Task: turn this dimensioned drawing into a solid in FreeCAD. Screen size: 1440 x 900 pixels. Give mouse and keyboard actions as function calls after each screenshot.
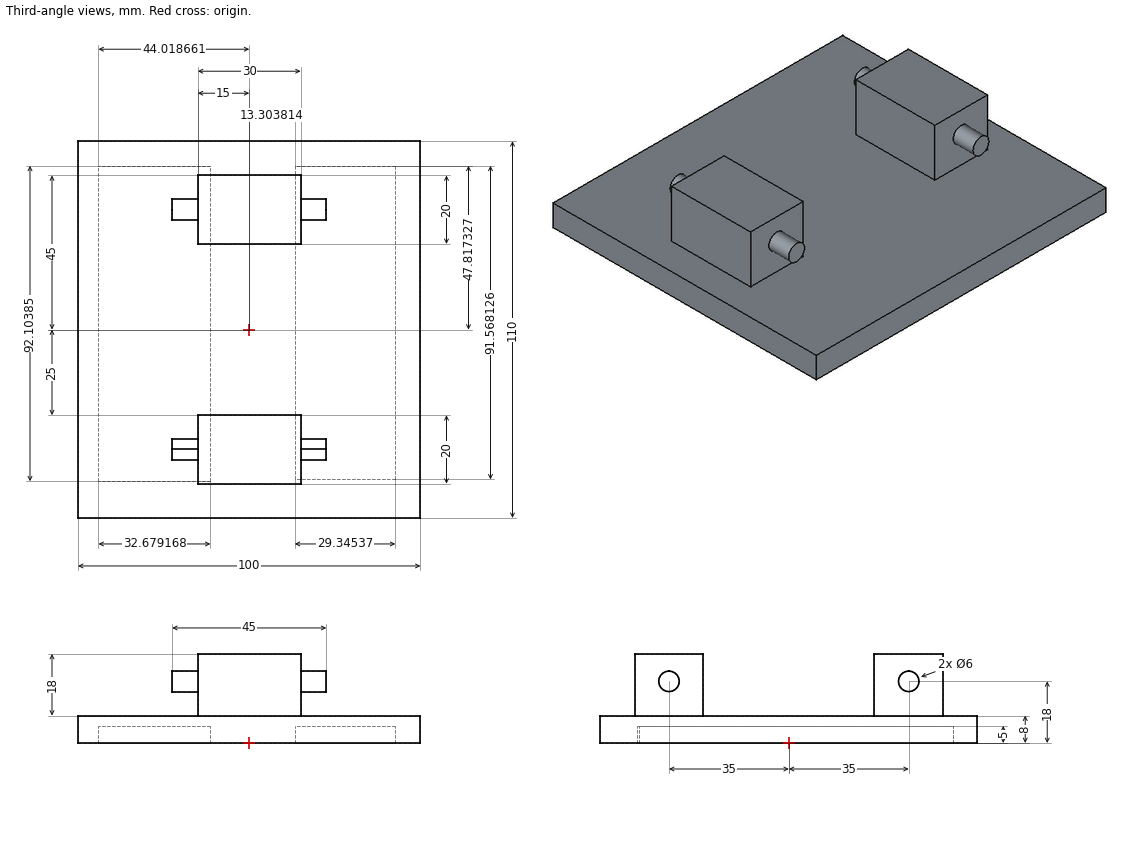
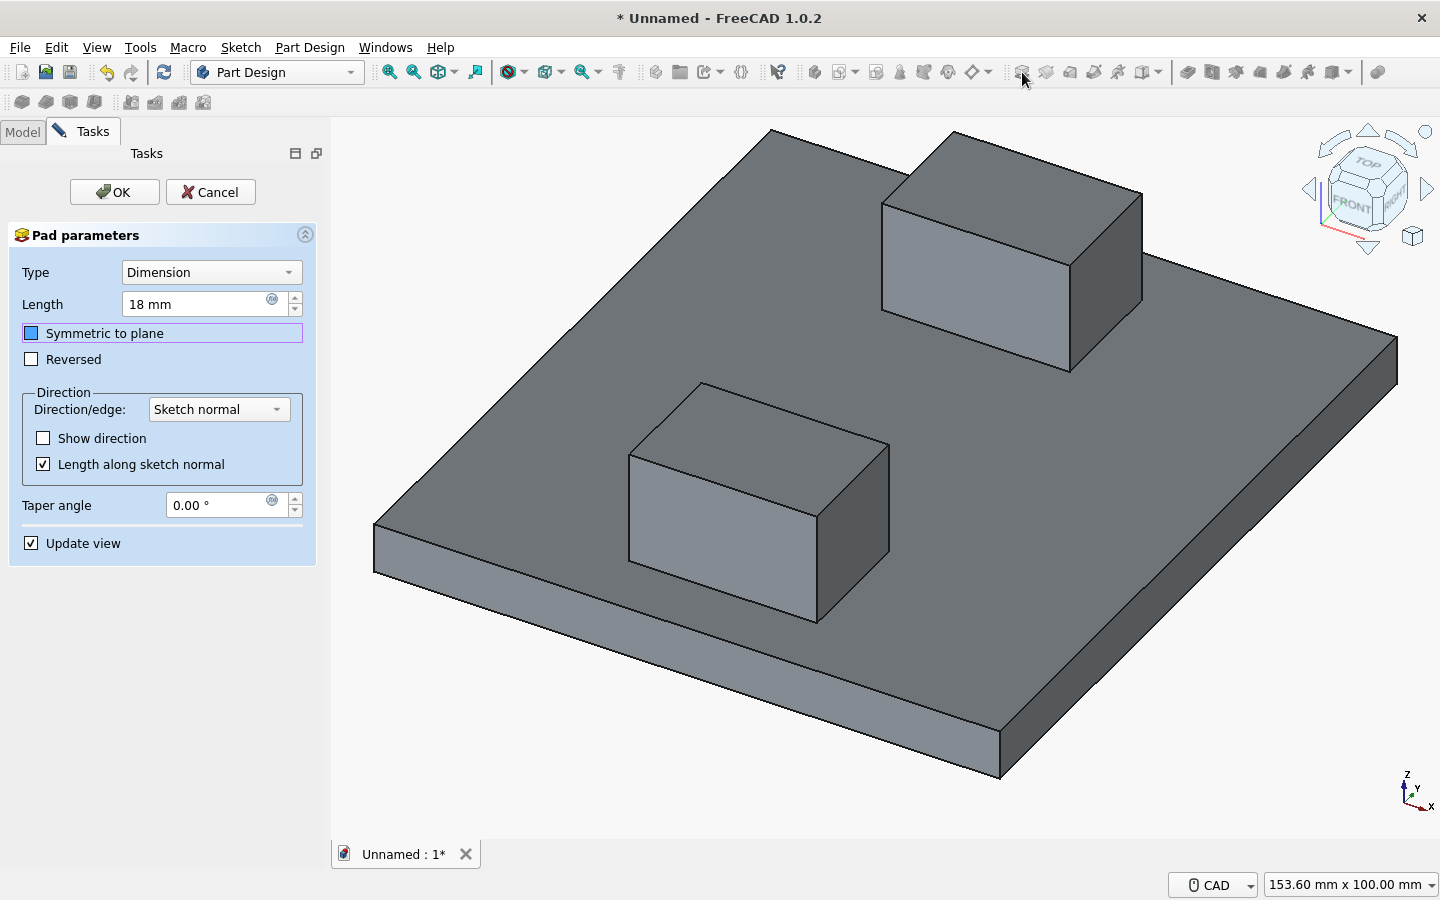
click(115, 192)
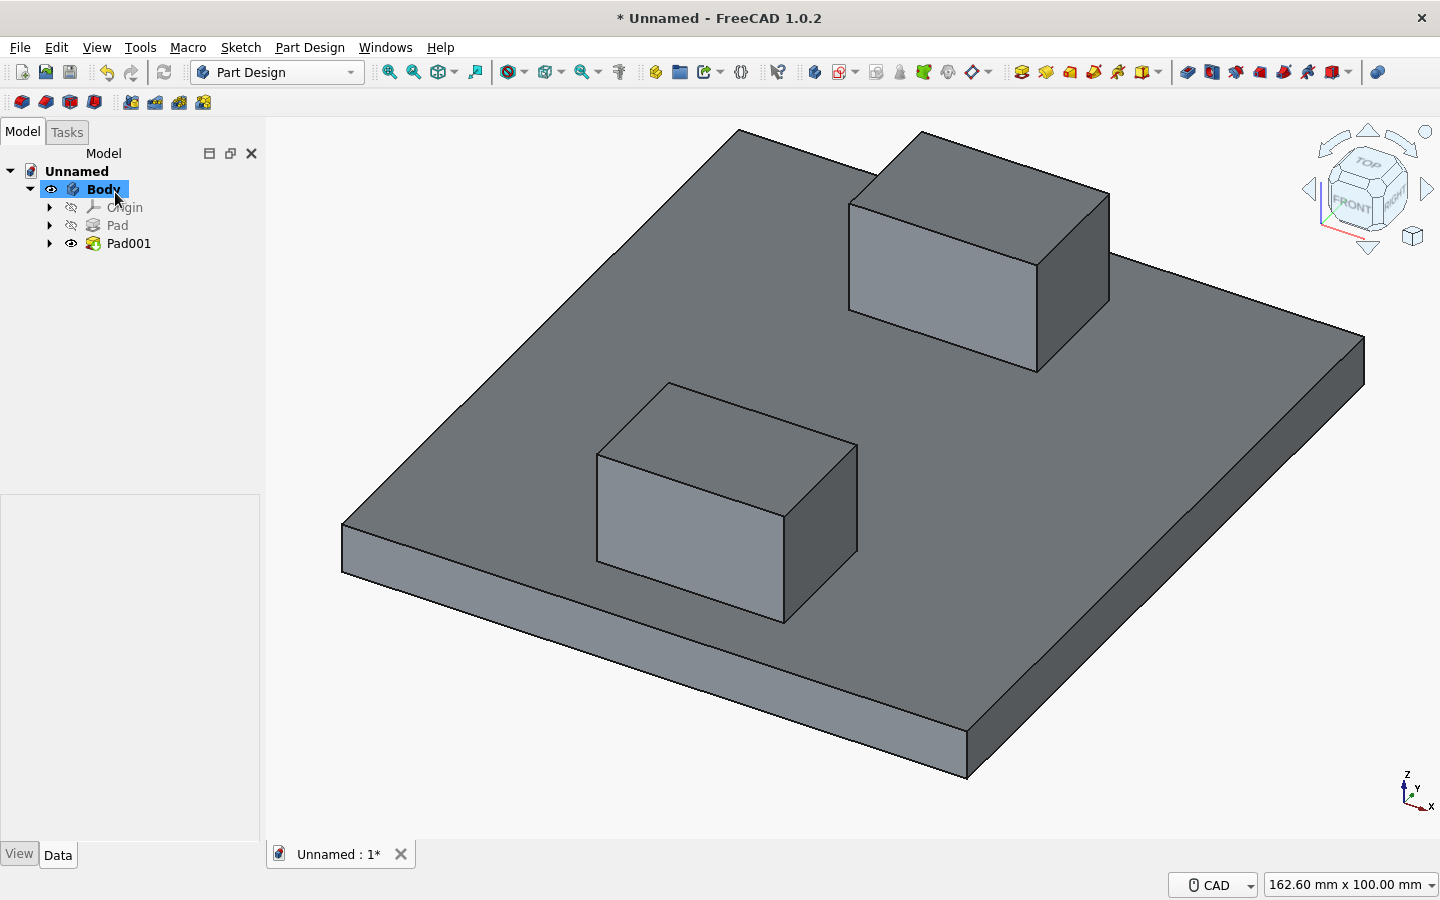
key(v)
key(f)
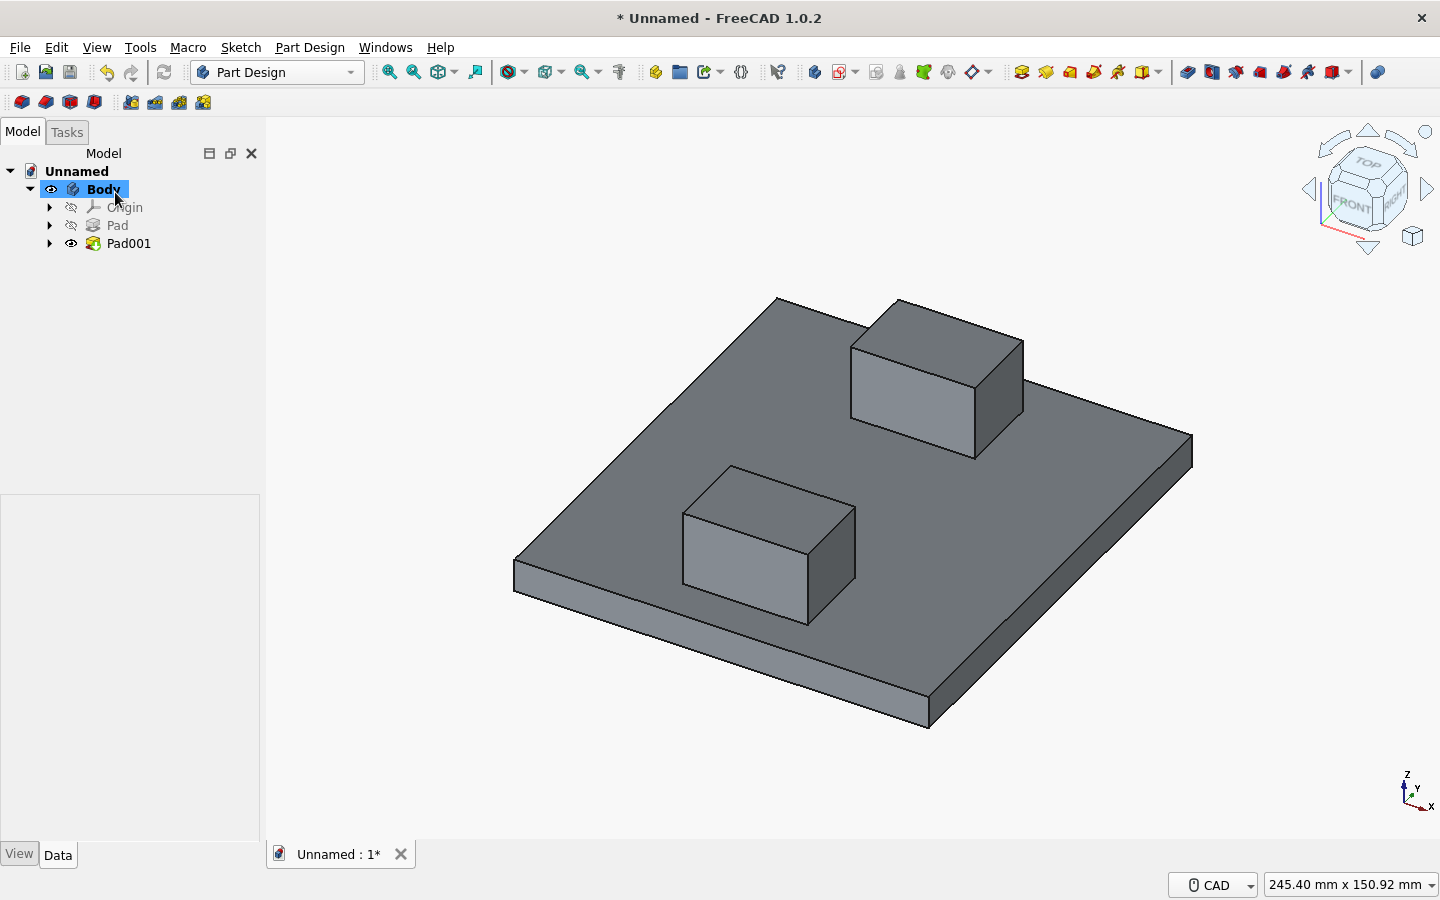
click(840, 72)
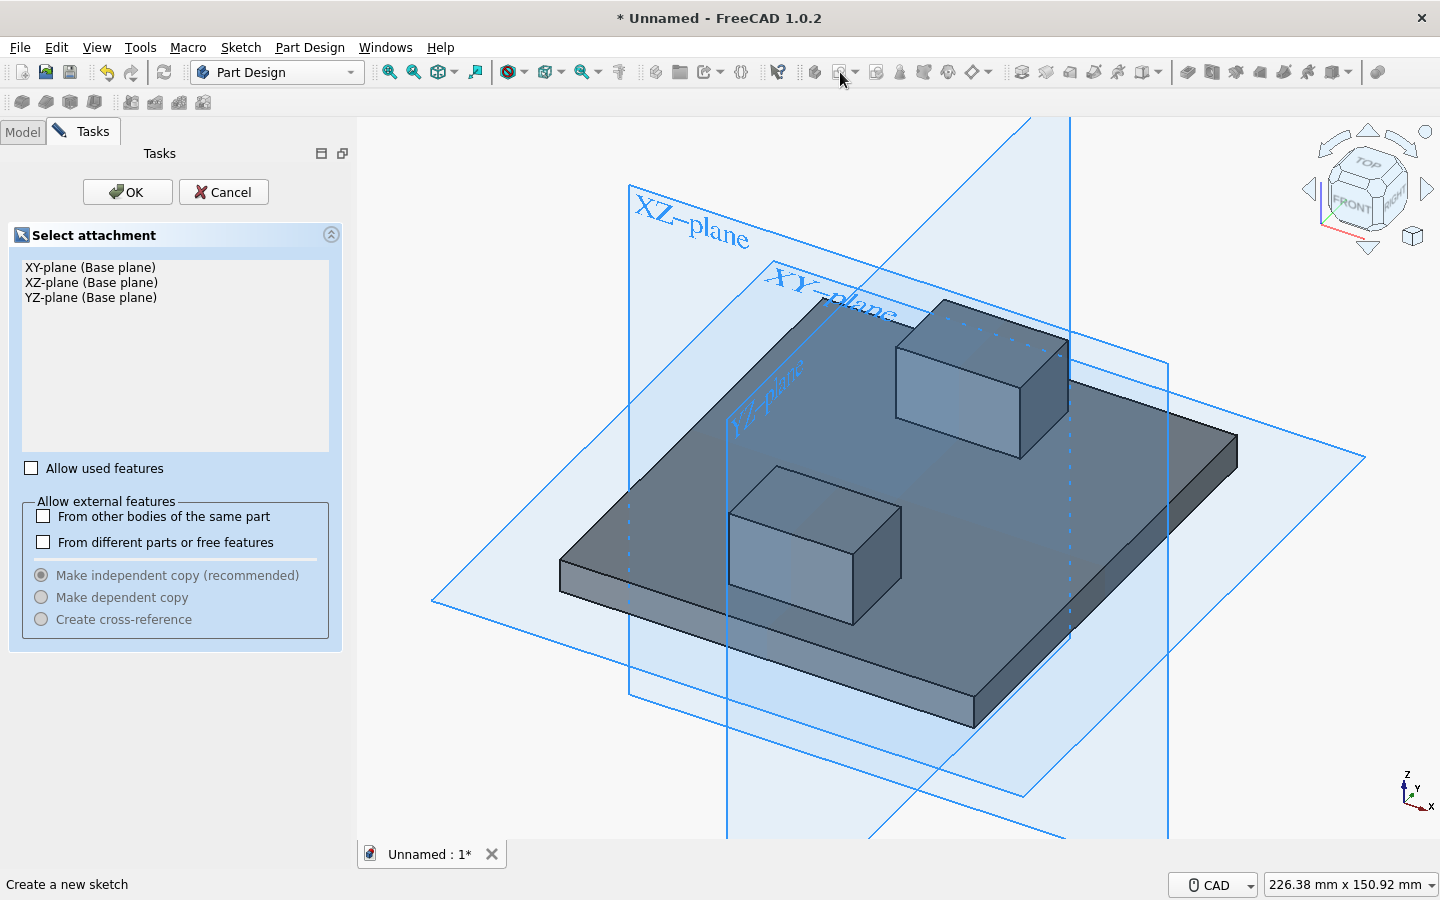
click(82, 268)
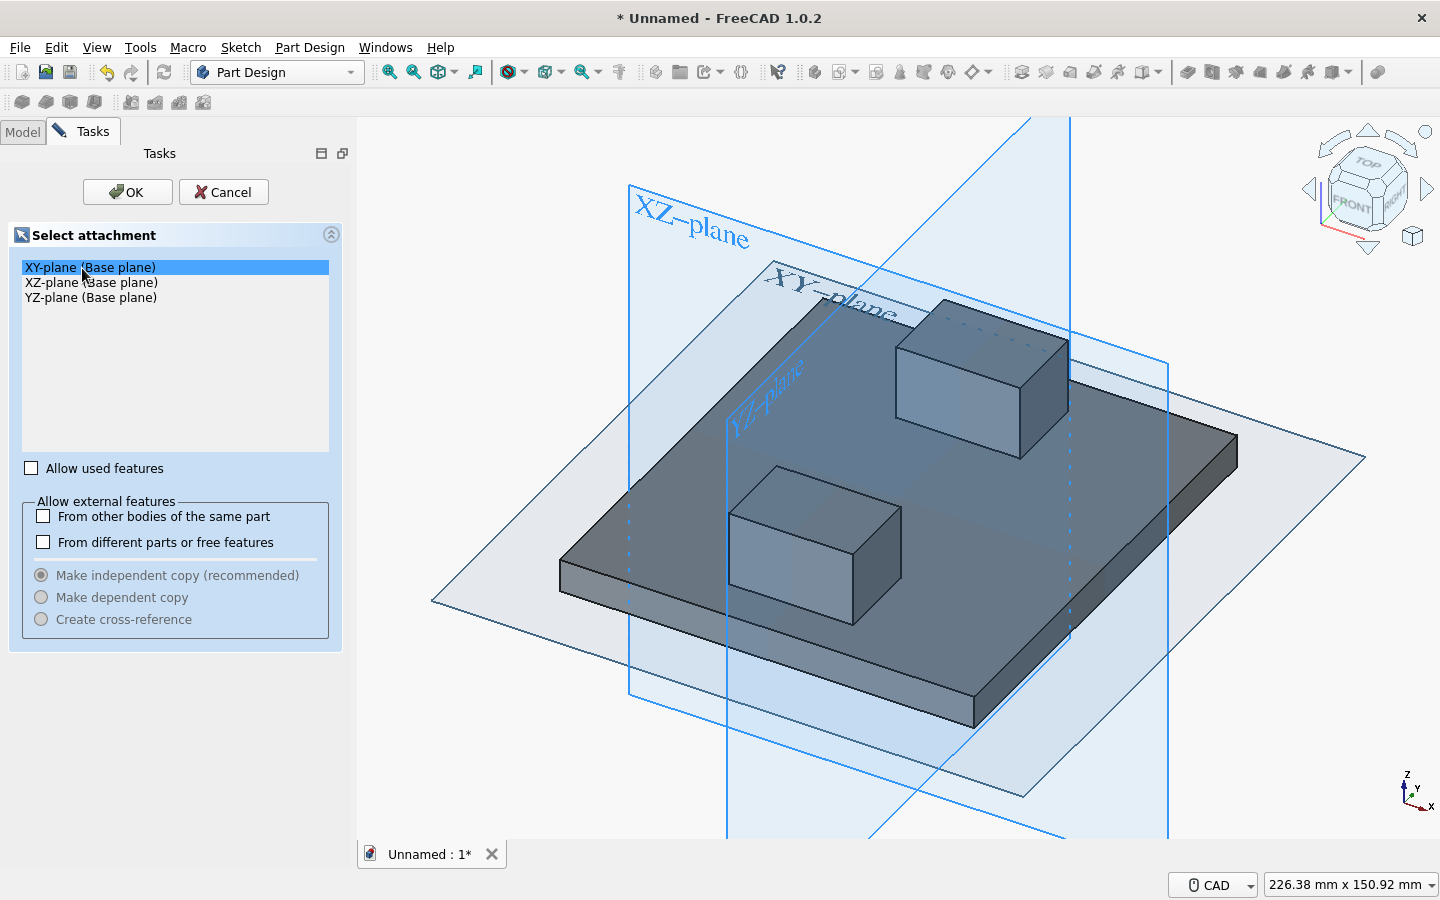
click(128, 192)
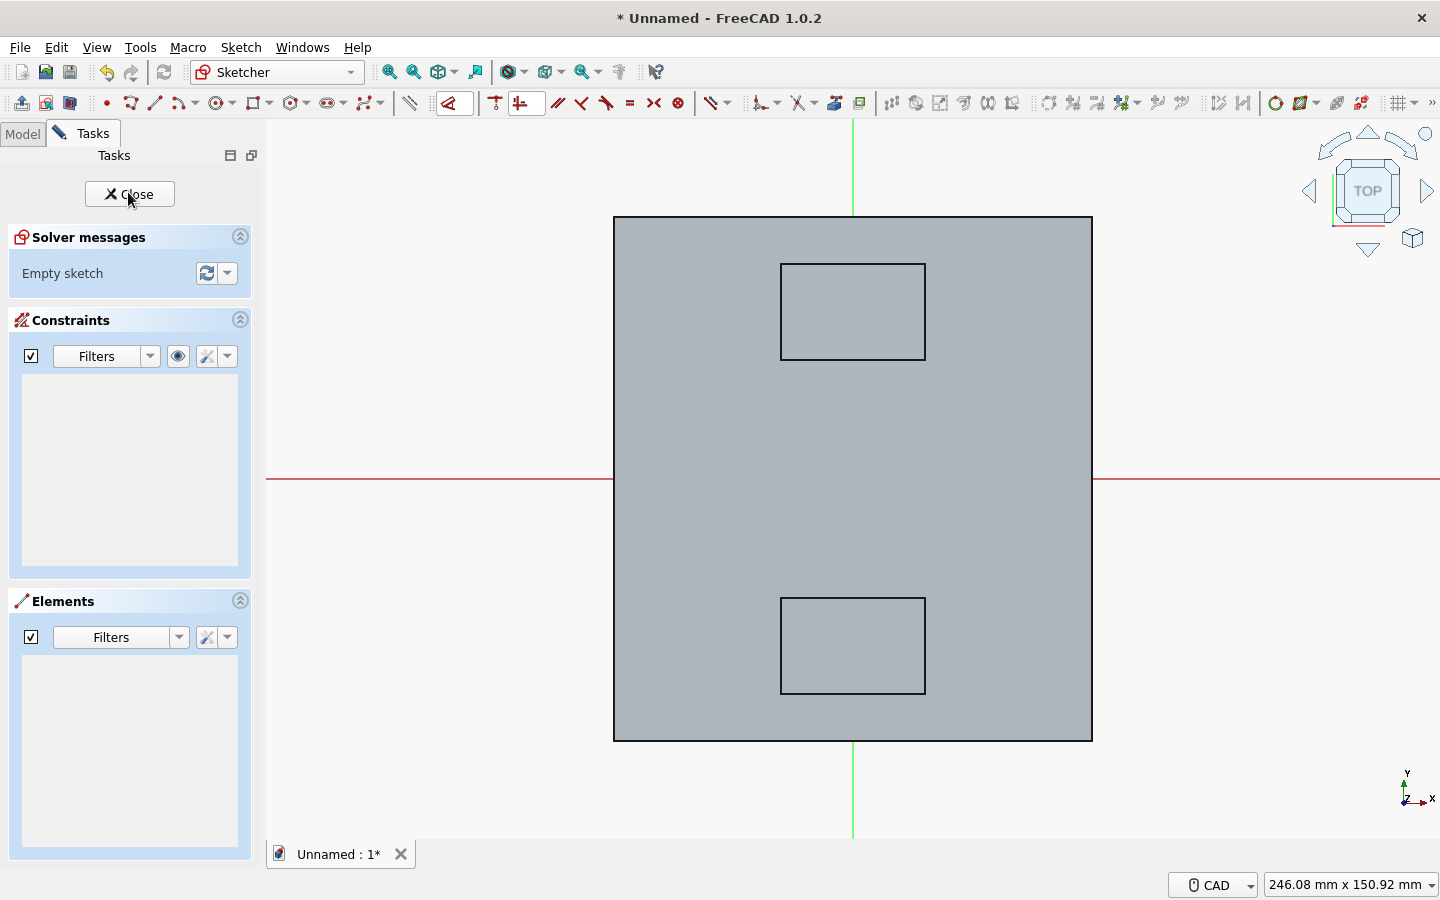
key(q)
key(s)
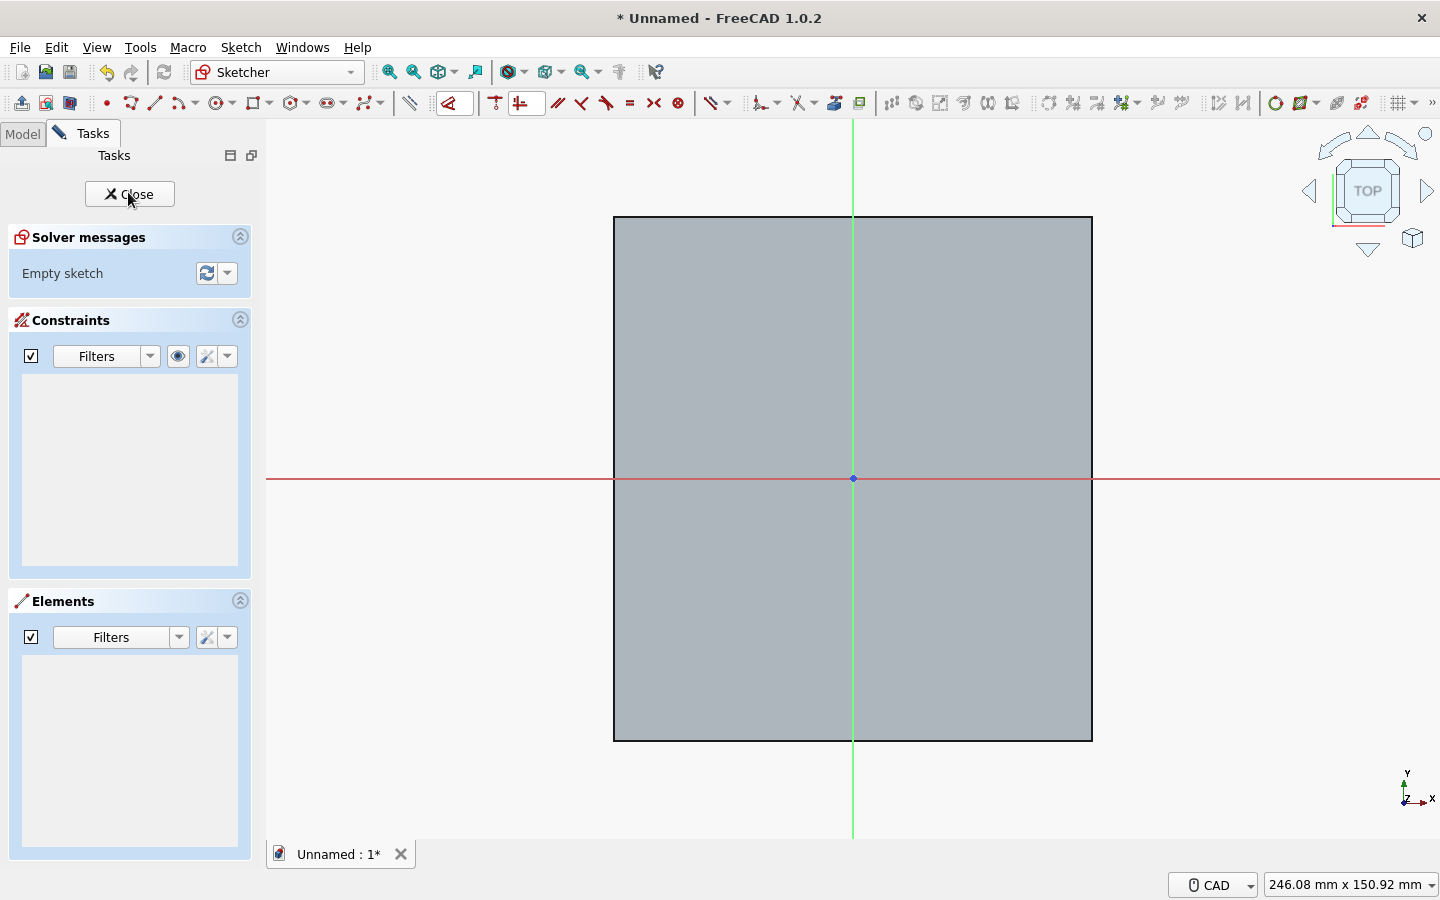
key(g)
key(r)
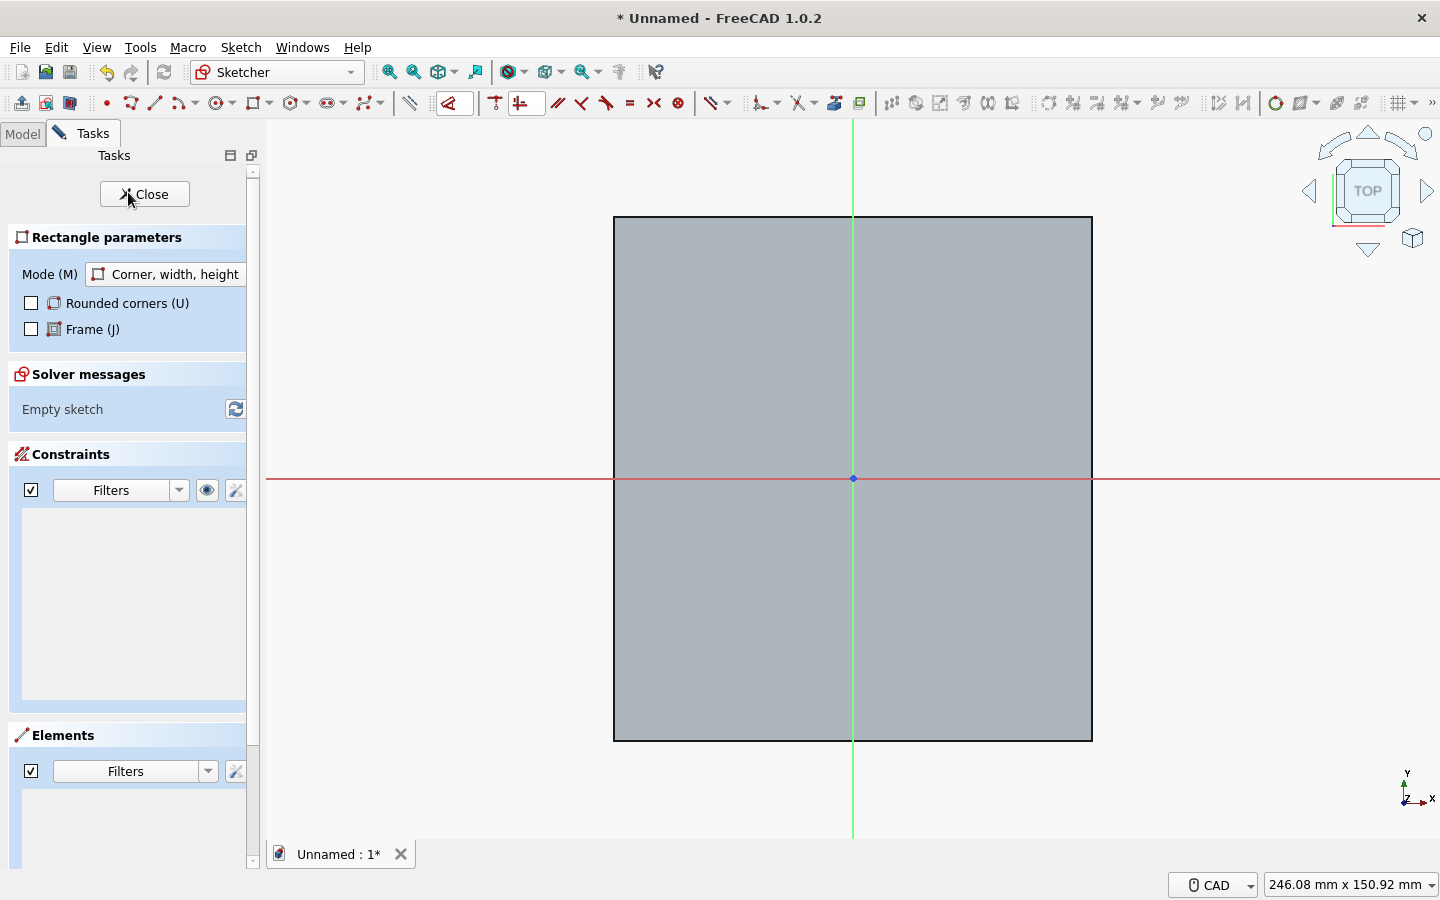
click(916, 251)
move(1056, 688)